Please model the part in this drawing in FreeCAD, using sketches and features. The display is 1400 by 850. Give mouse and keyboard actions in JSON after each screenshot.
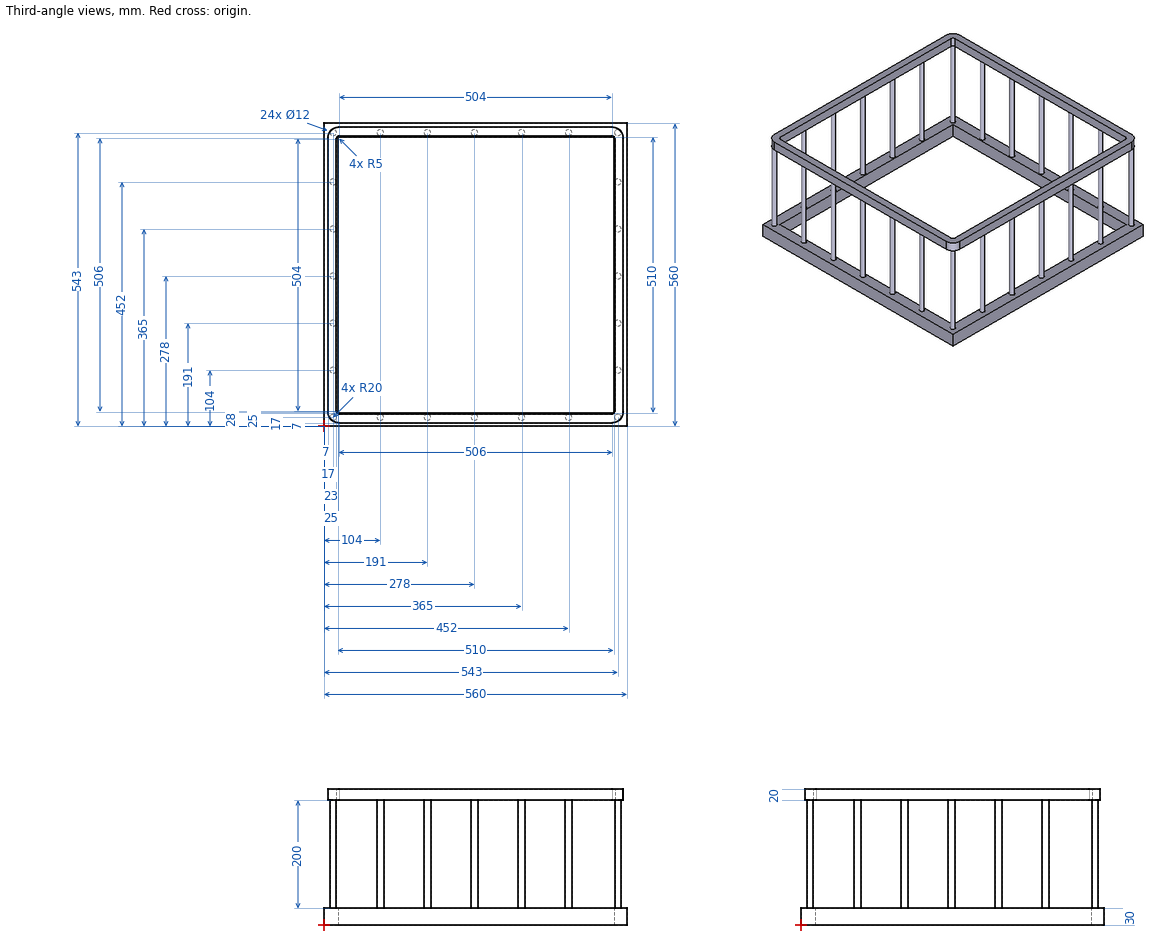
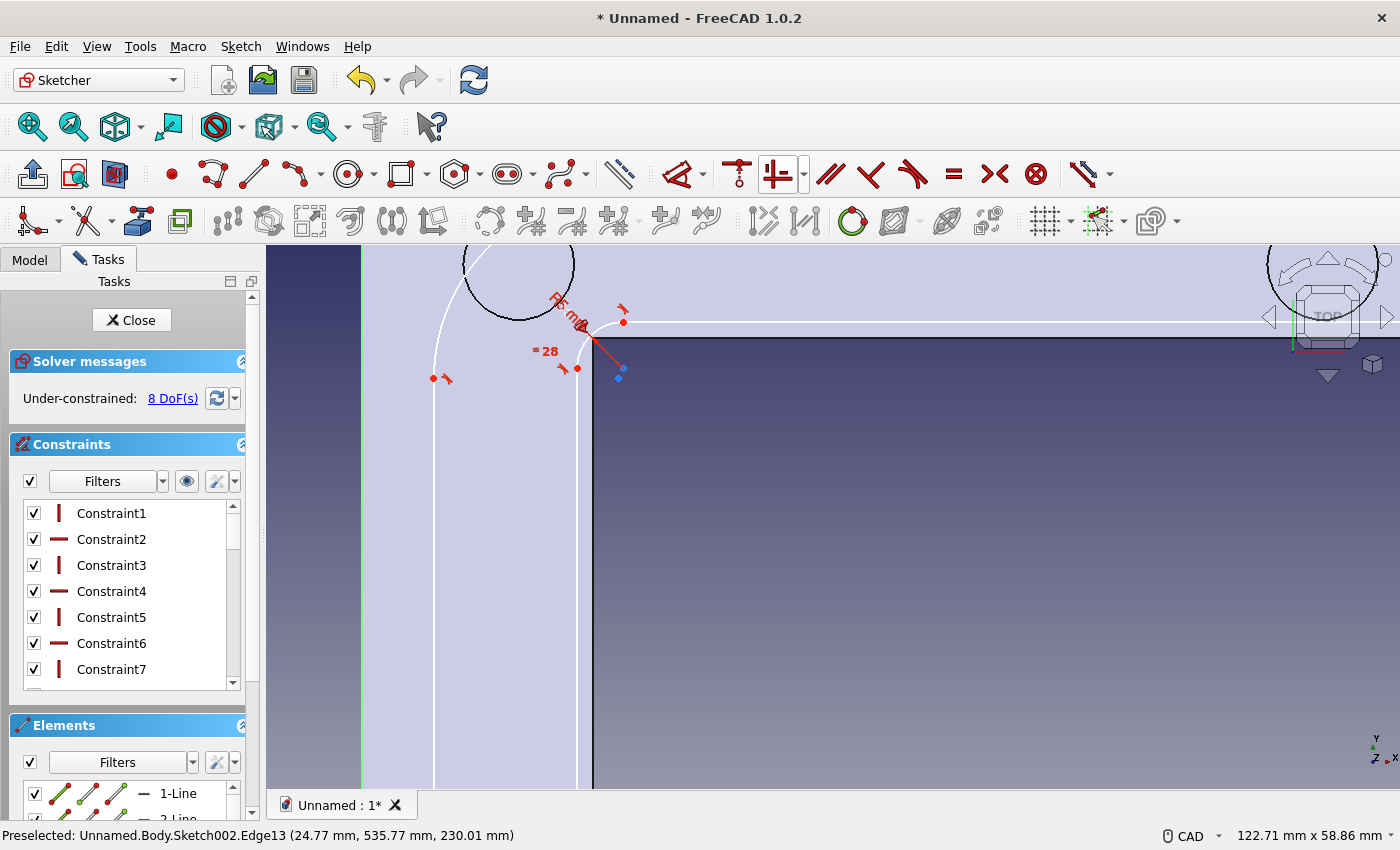
{"action": "left_click", "coordinate": [434, 378]}
{"action": "left_click", "coordinate": [398, 344]}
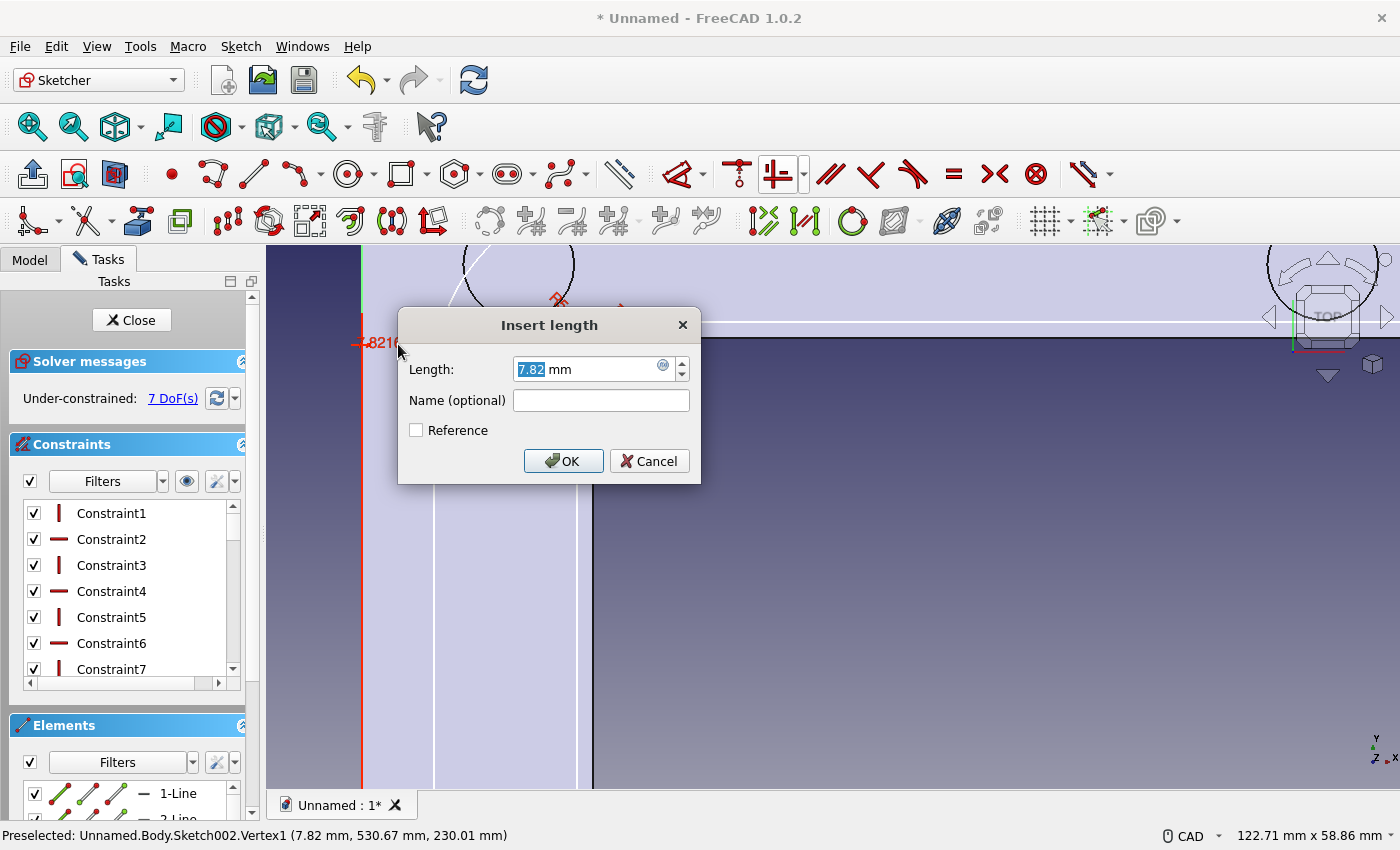
{"action": "type", "text": "7"}
{"action": "key", "text": "Return"}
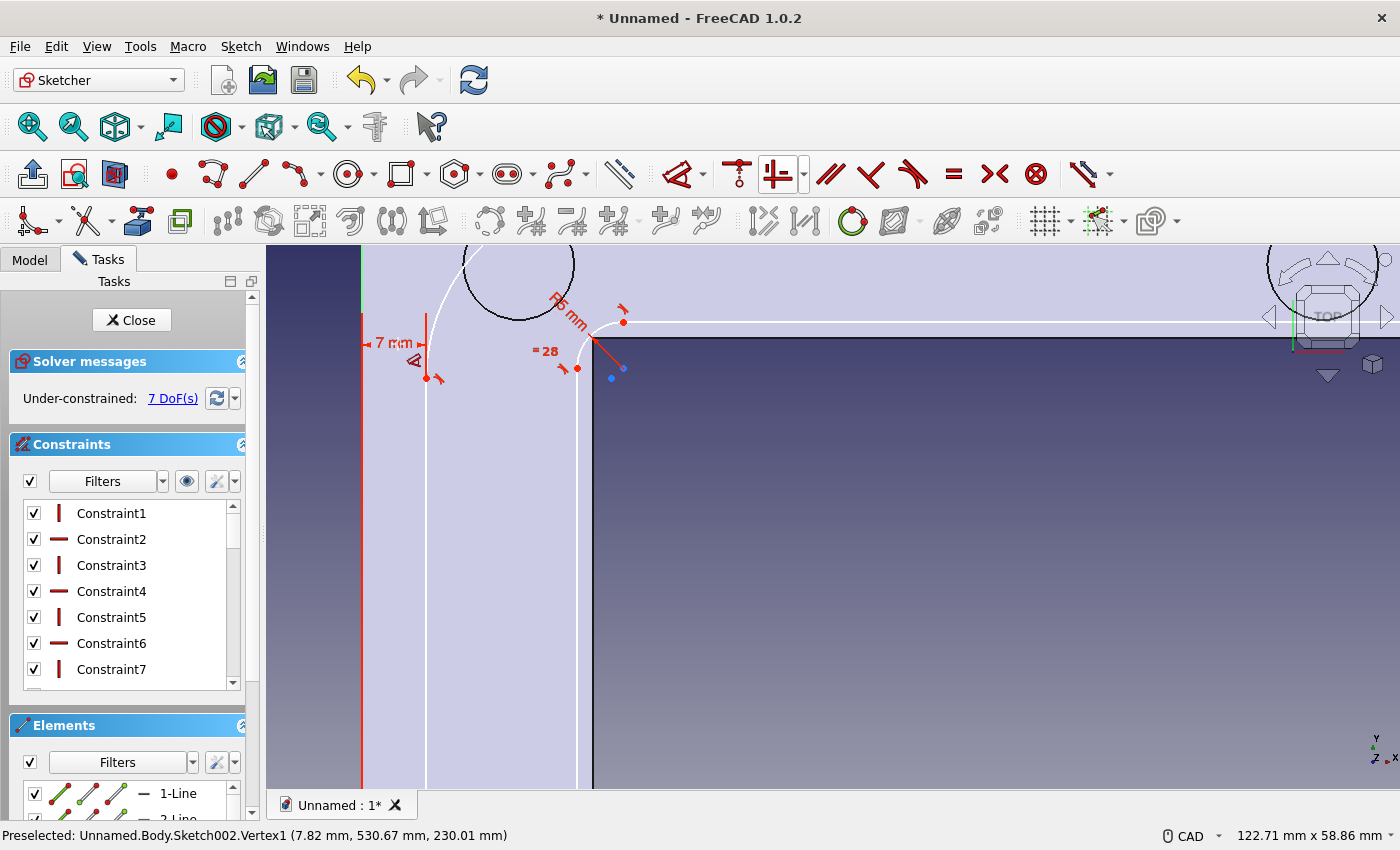
{"action": "scroll", "coordinate": [592, 340], "scroll_direction": "down", "scroll_amount": 13}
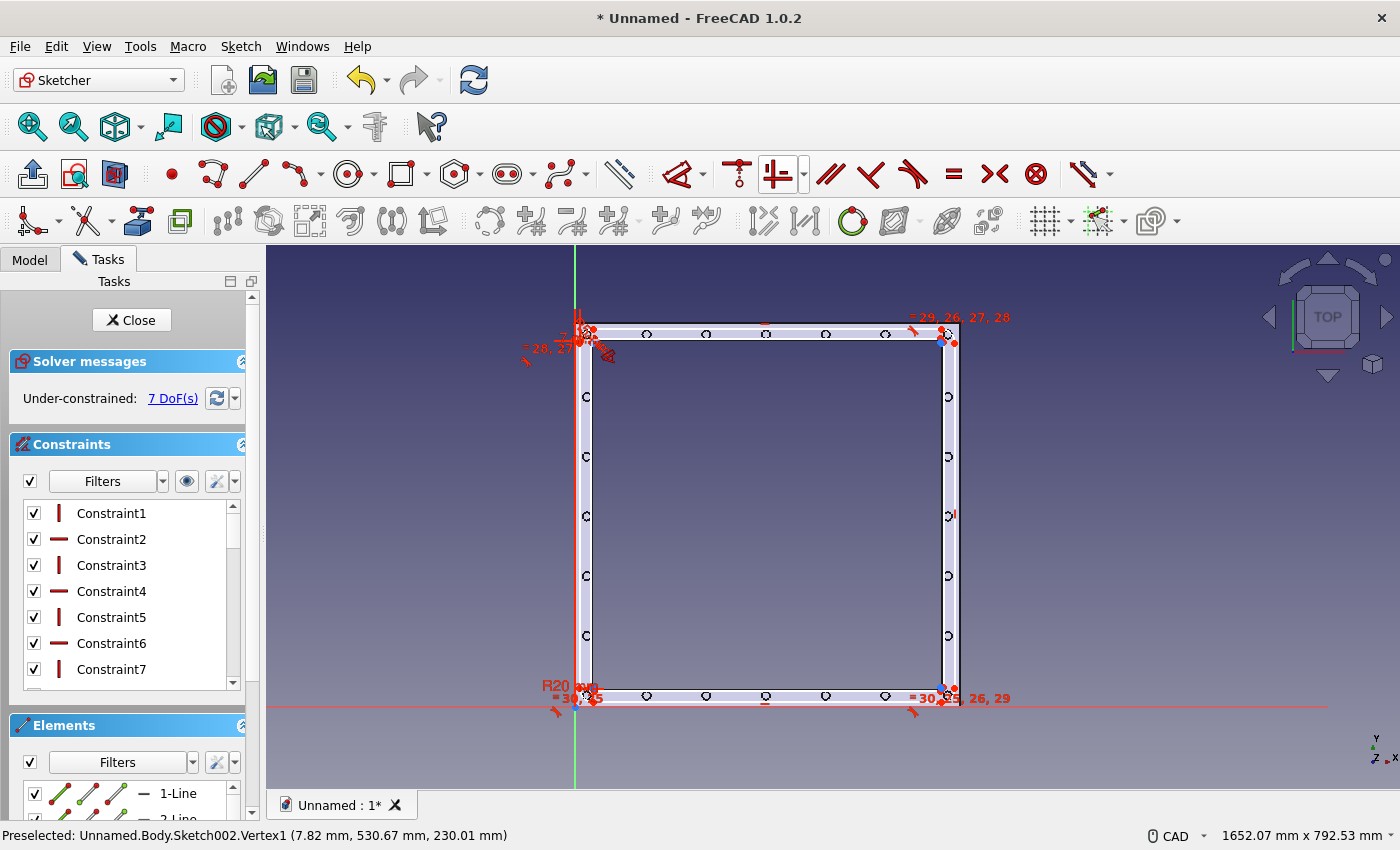
{"action": "scroll", "coordinate": [594, 702], "scroll_direction": "up", "scroll_amount": 11}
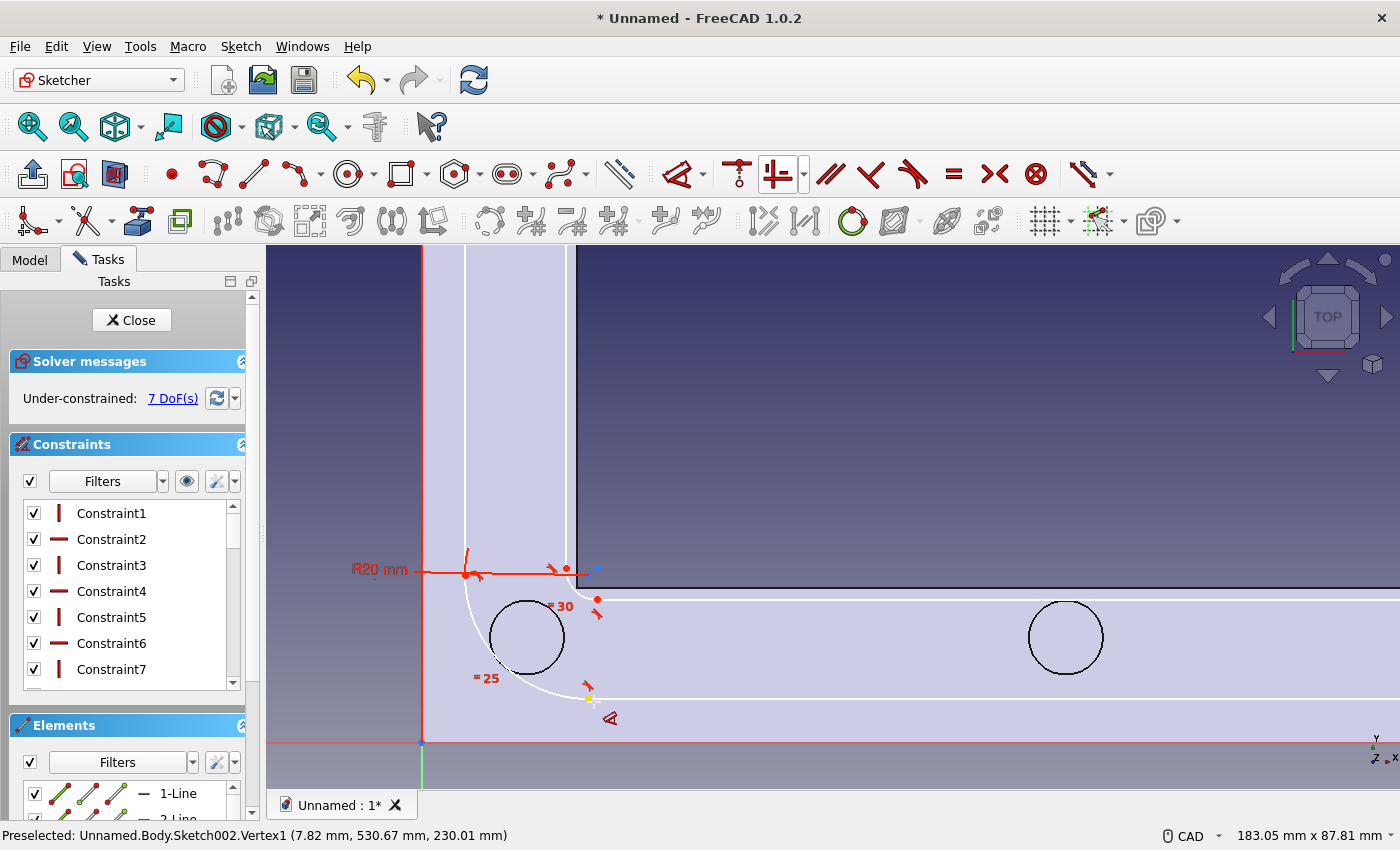
{"action": "left_click", "coordinate": [589, 699]}
{"action": "left_click", "coordinate": [388, 721]}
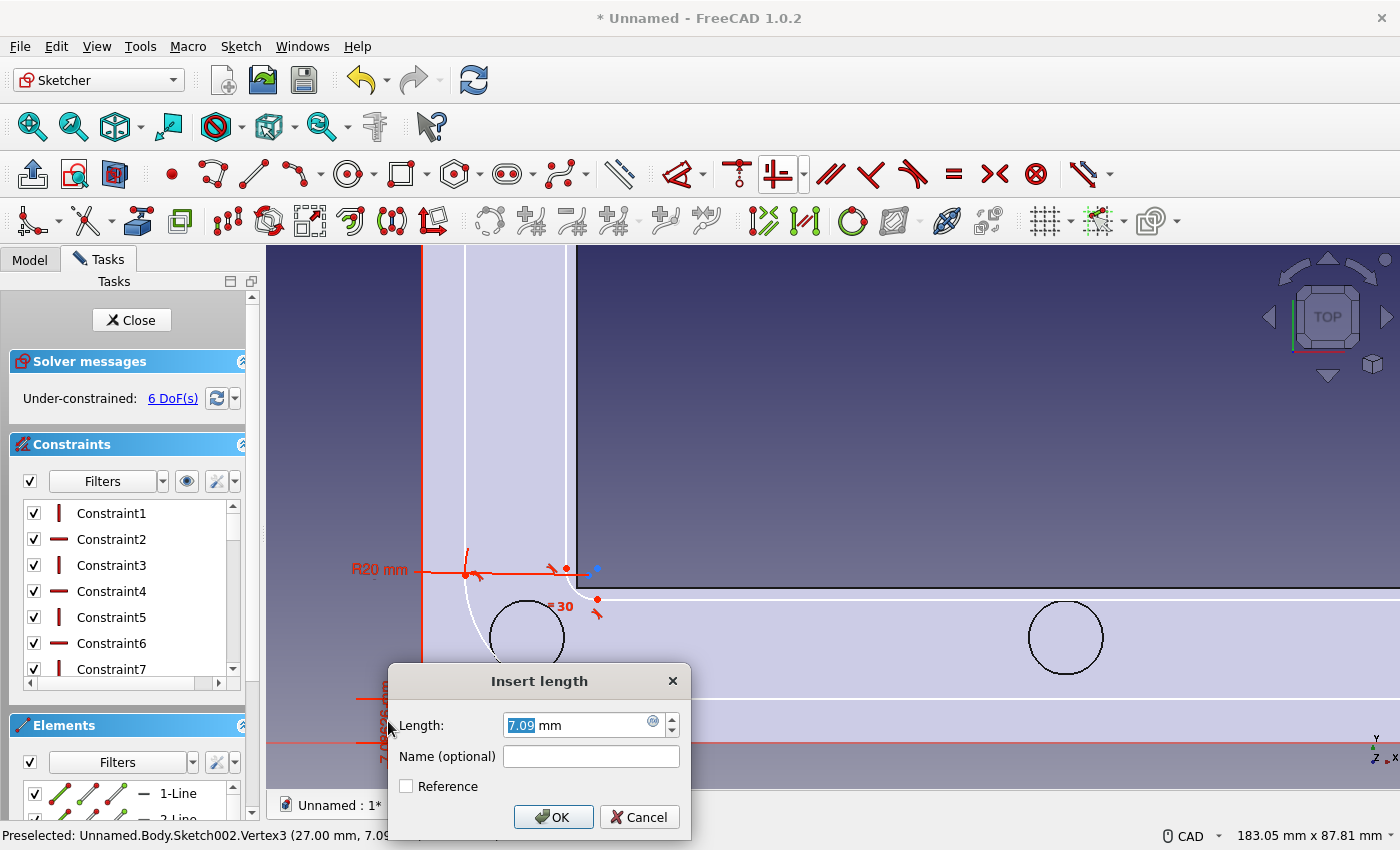
{"action": "type", "text": "7"}
{"action": "key", "text": "Return"}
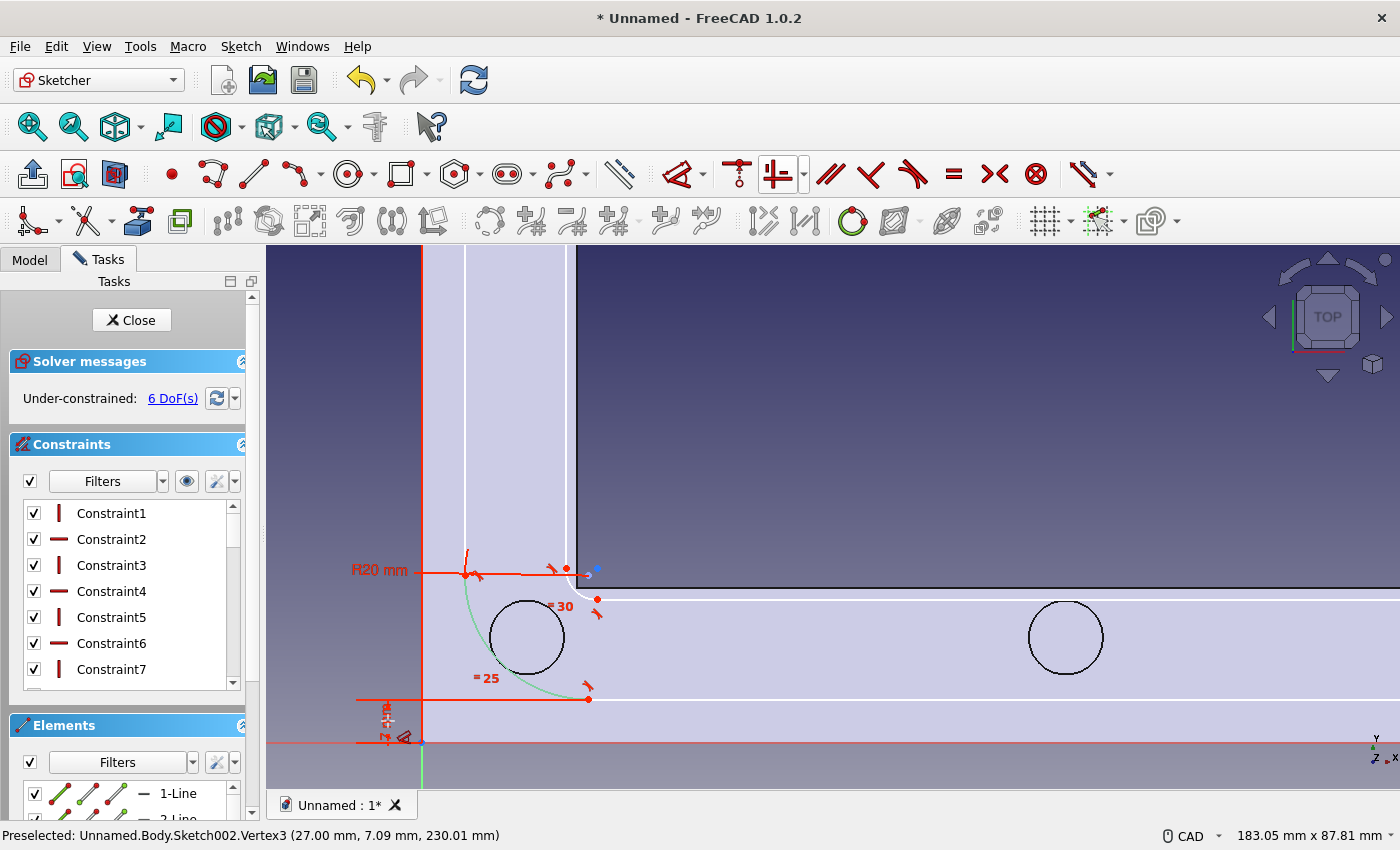
{"action": "scroll", "coordinate": [594, 702], "scroll_direction": "down", "scroll_amount": 11}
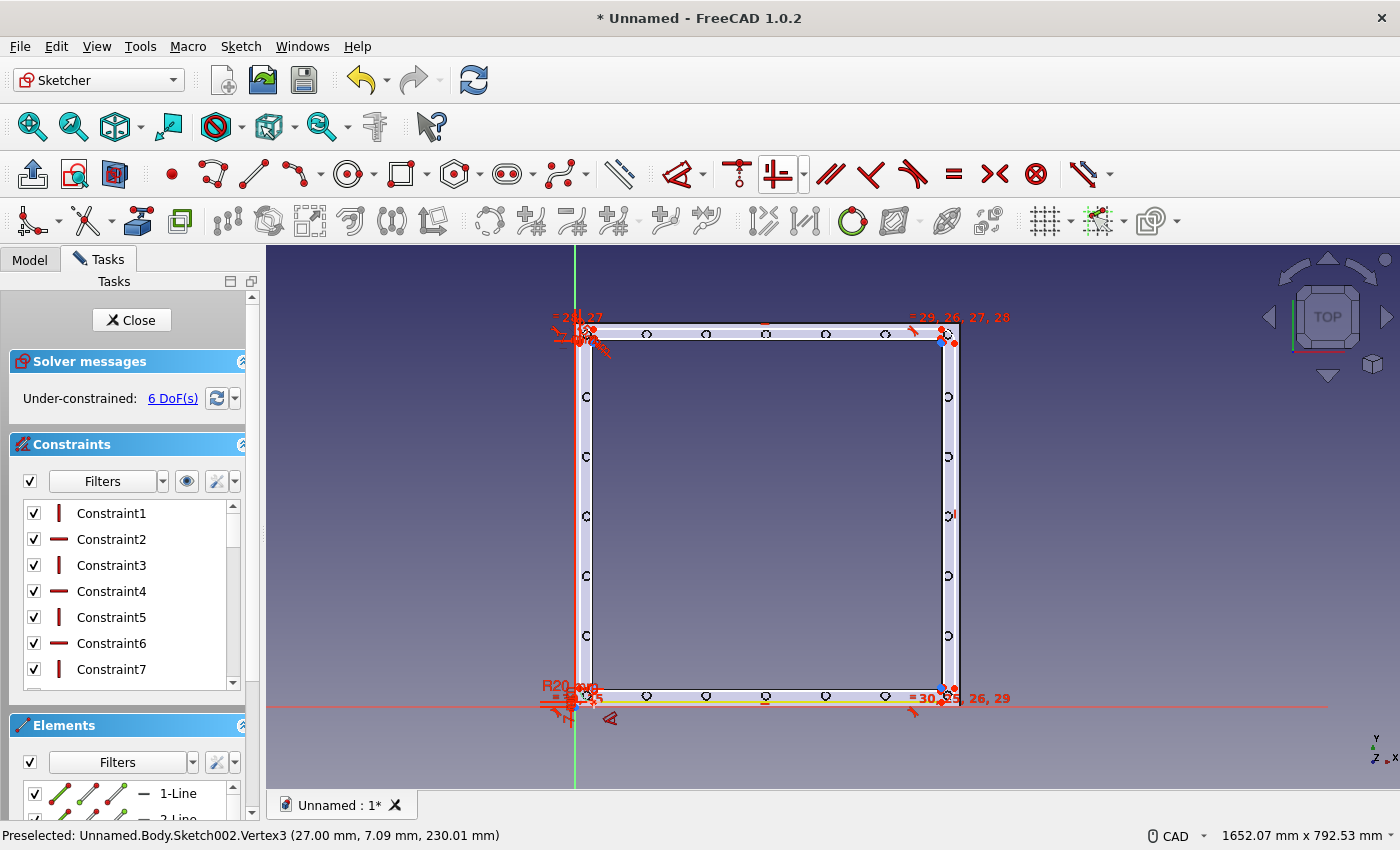
{"action": "scroll", "coordinate": [580, 447], "scroll_direction": "up", "scroll_amount": 6}